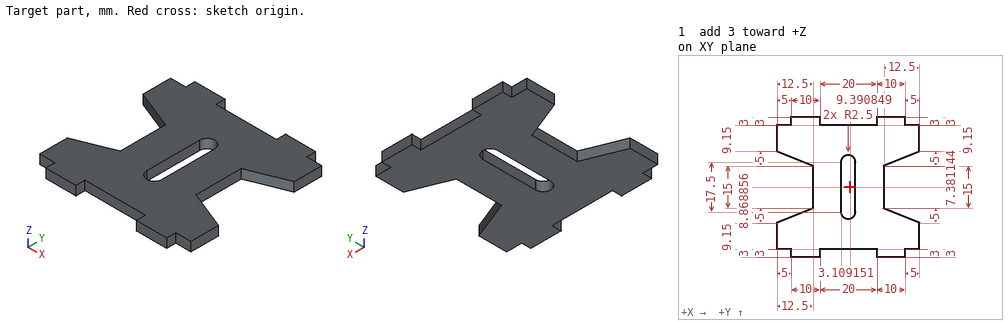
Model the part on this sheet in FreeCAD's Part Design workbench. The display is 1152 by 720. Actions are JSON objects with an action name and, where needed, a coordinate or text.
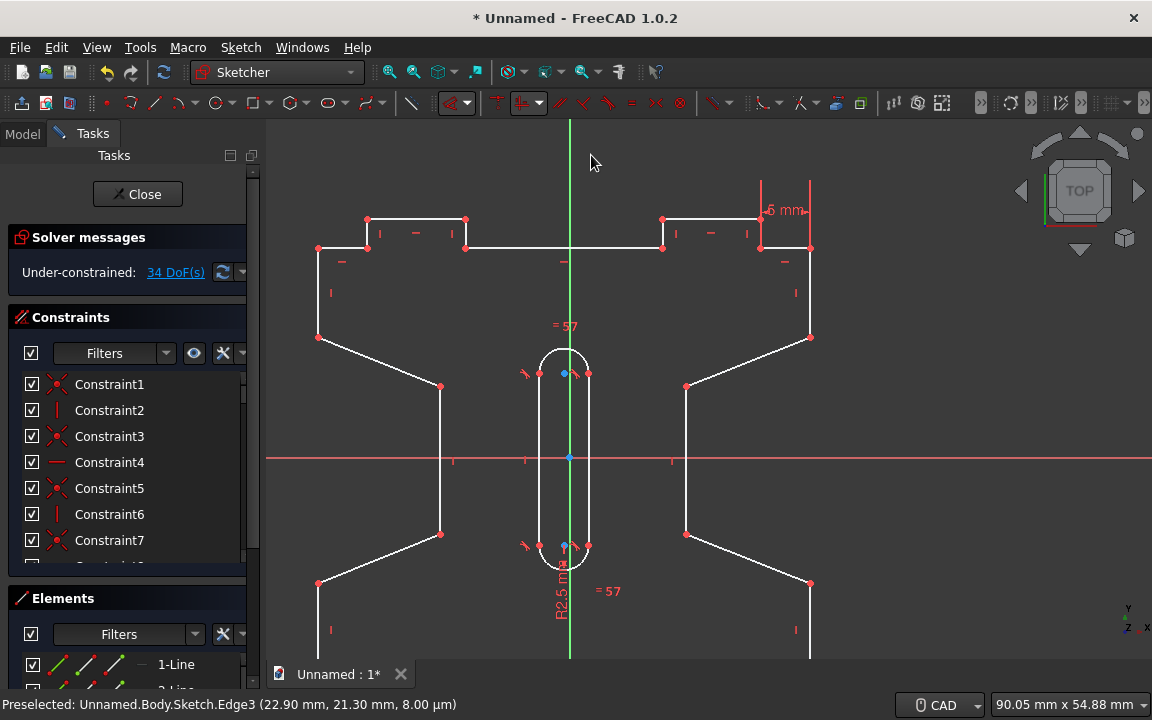
{"action": "scroll", "coordinate": [761, 237], "scroll_direction": "up", "scroll_amount": 2}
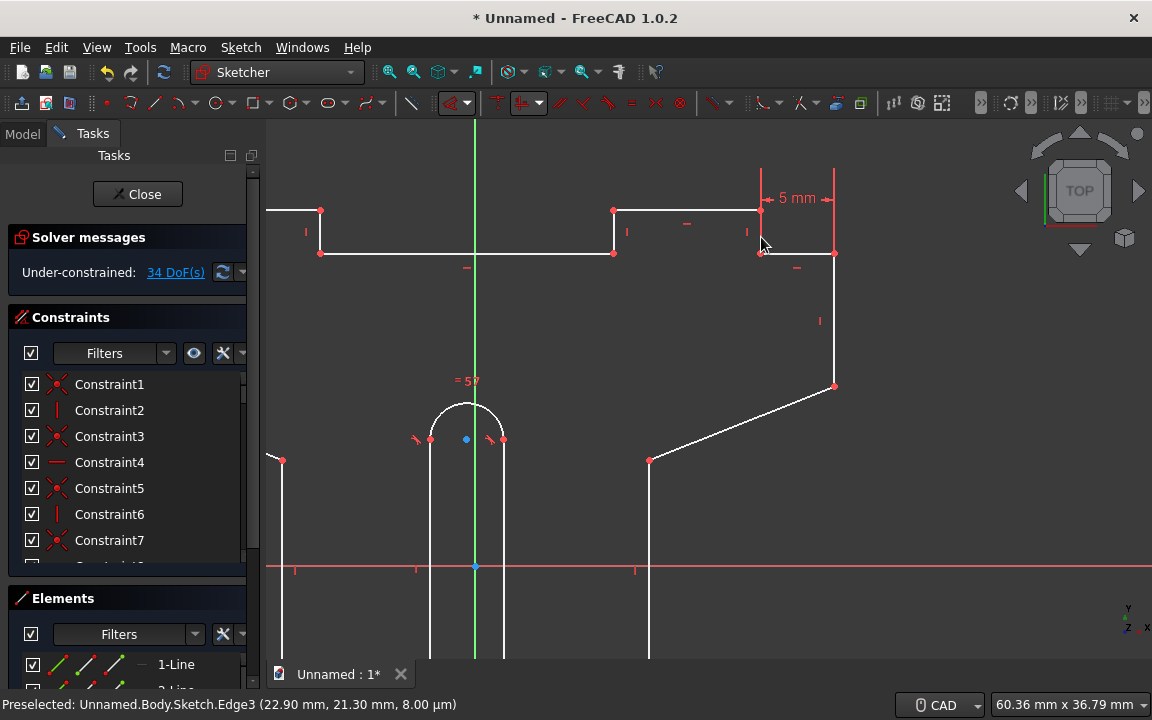
{"action": "left_click", "coordinate": [761, 236]}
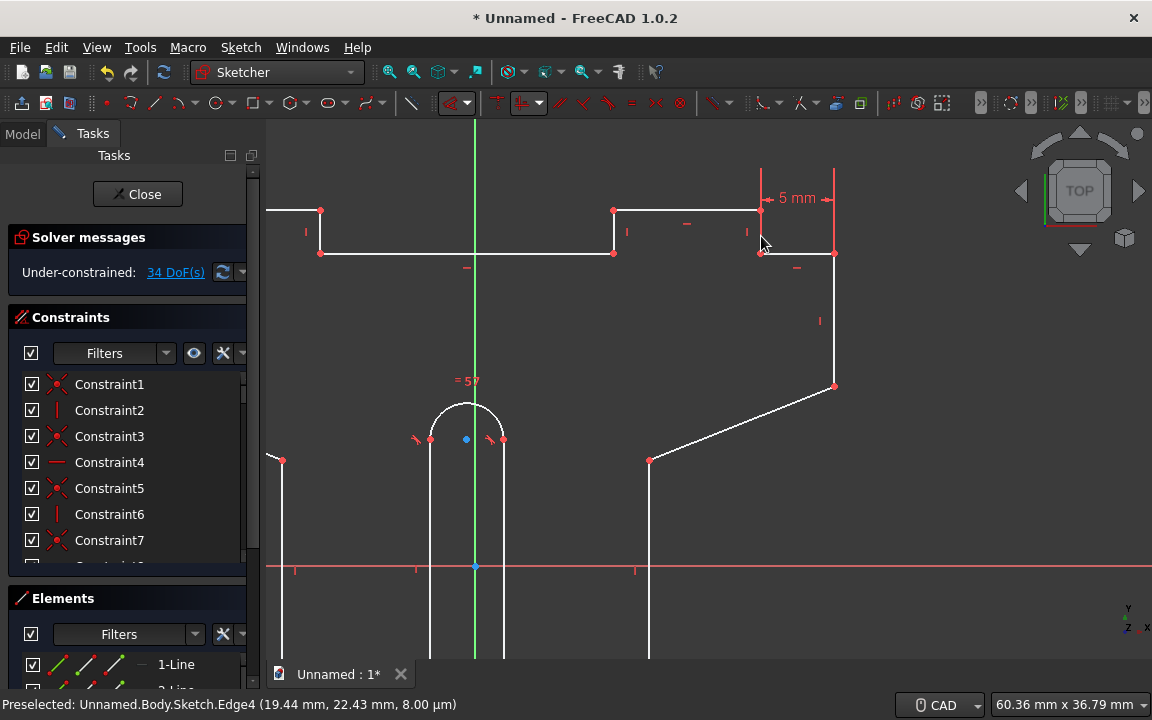
{"action": "left_click", "coordinate": [470, 104]}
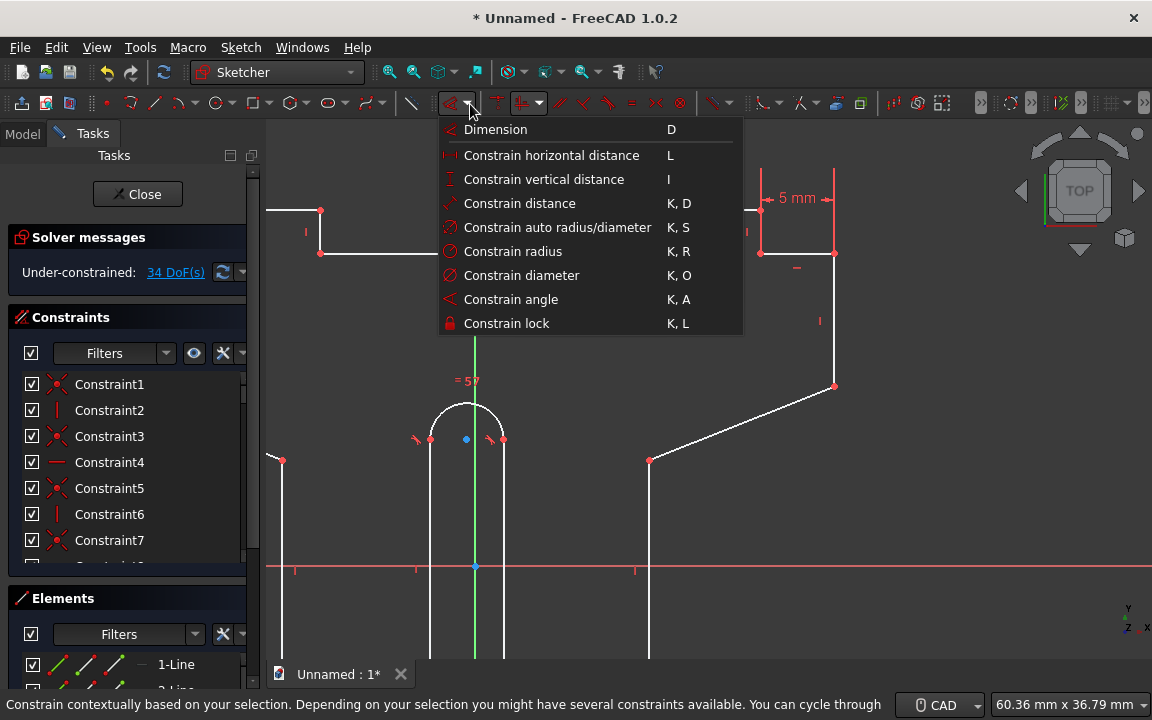
{"action": "left_click", "coordinate": [591, 179]}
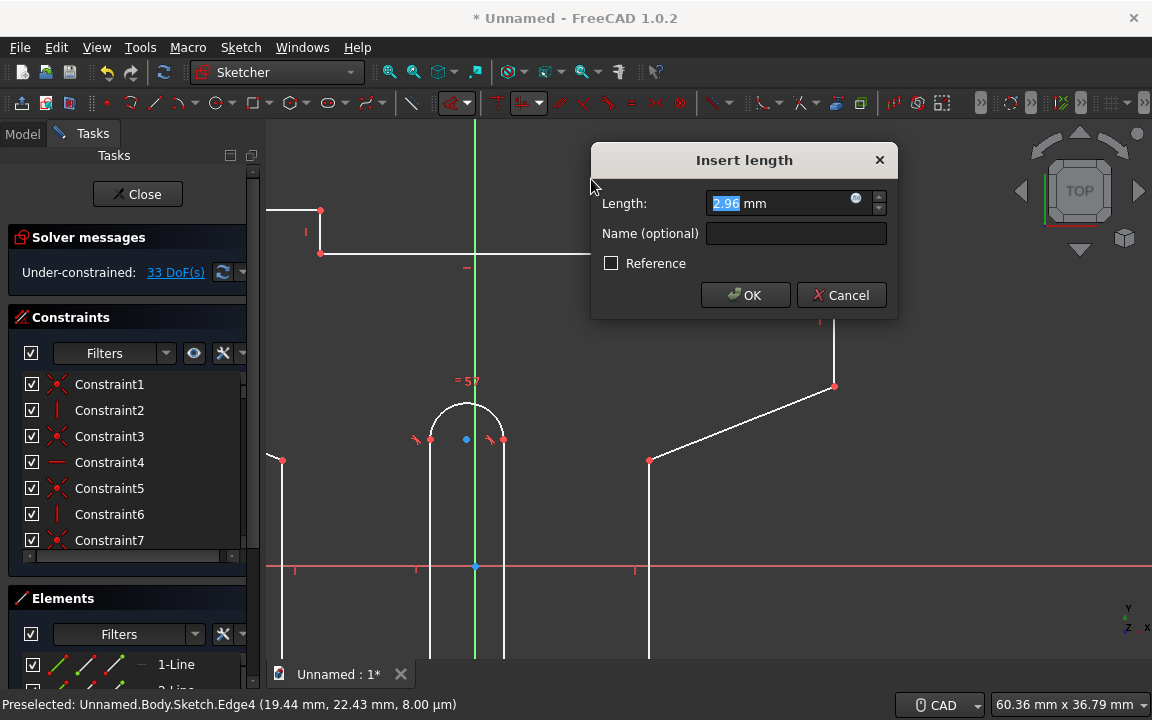
{"action": "type", "text": "3"}
{"action": "key", "text": "Return"}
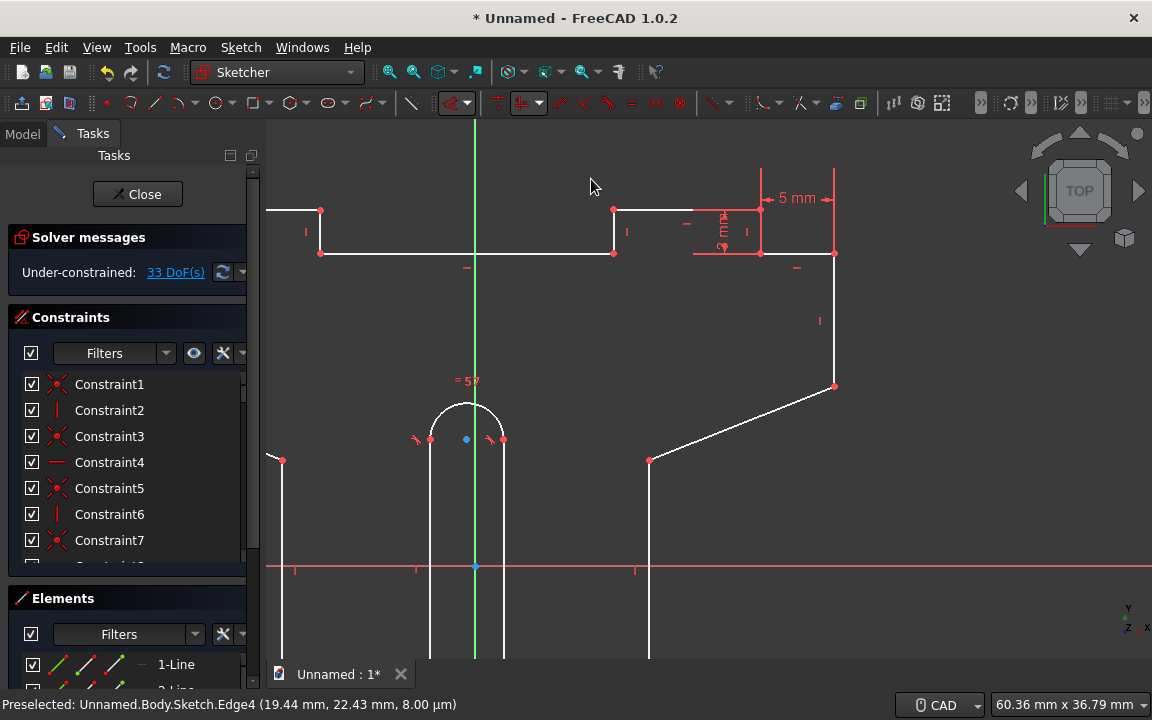
{"action": "left_click", "coordinate": [614, 223]}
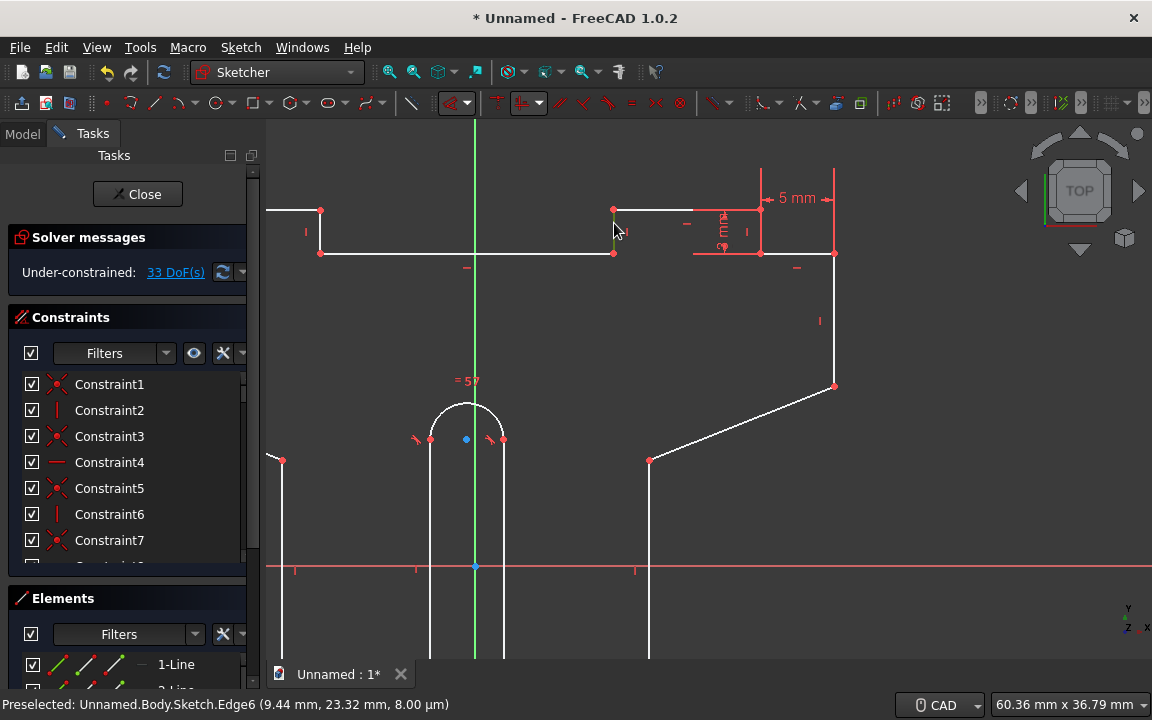
{"action": "key", "text": "i"}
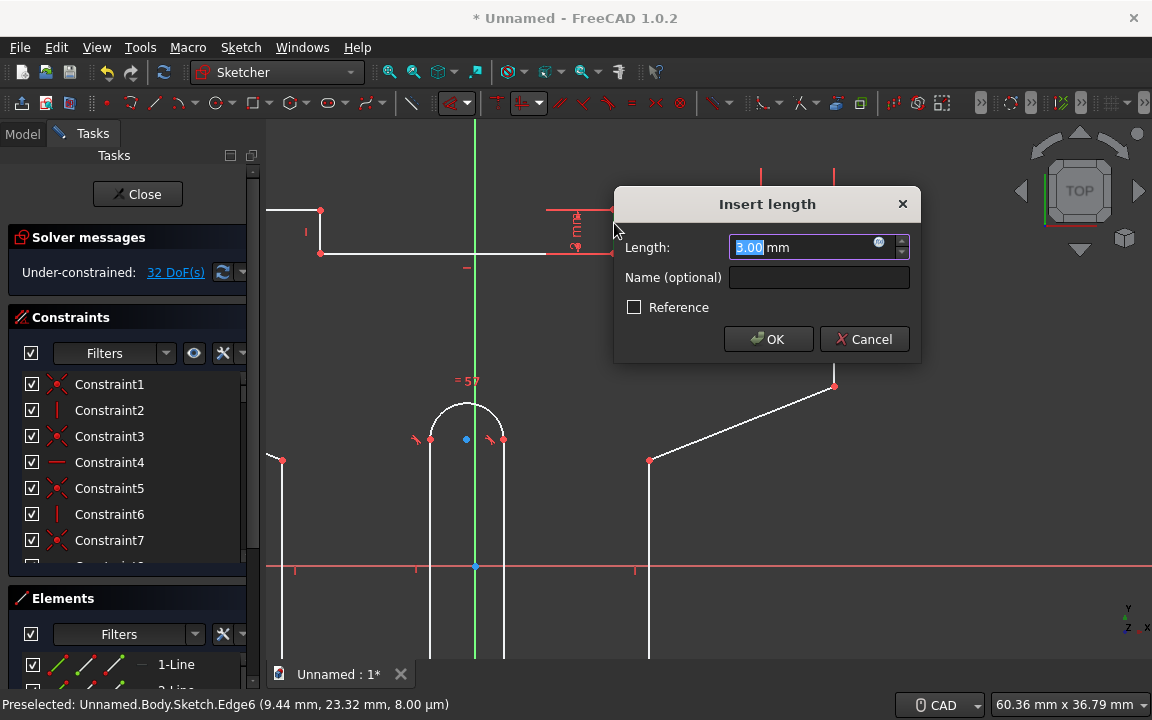
{"action": "type", "text": "3"}
{"action": "key", "text": "Return"}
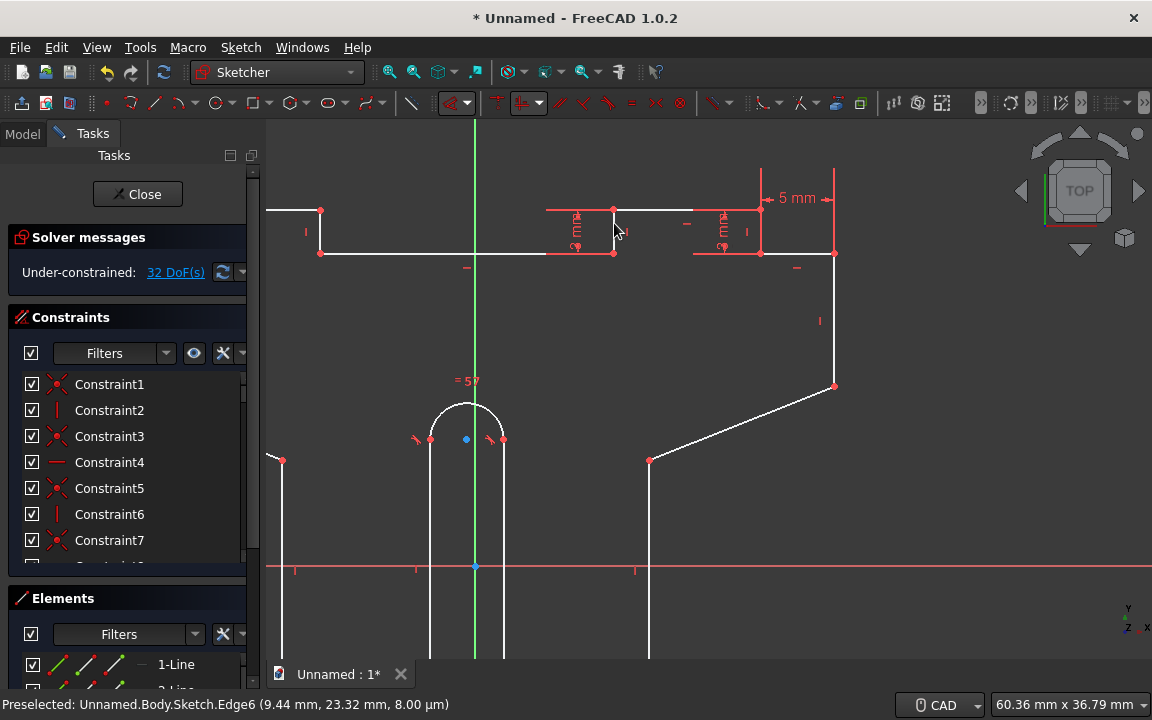
{"action": "left_click", "coordinate": [320, 241]}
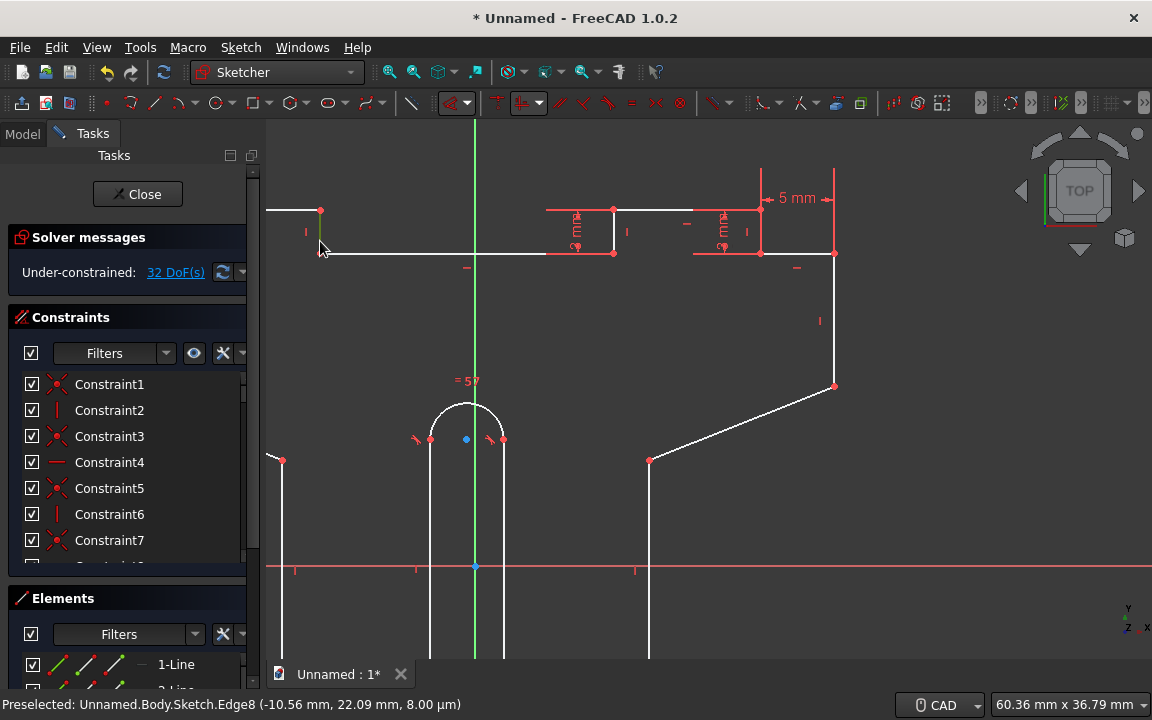
{"action": "key", "text": "i"}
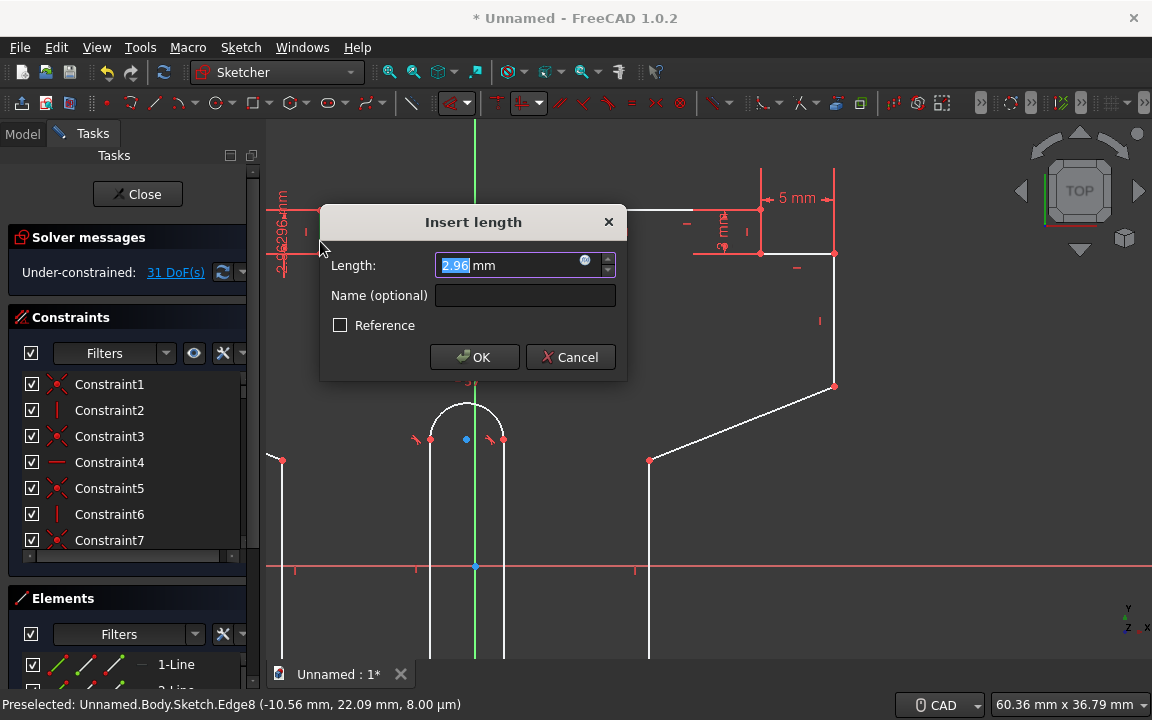
{"action": "type", "text": "3"}
{"action": "key", "text": "Return"}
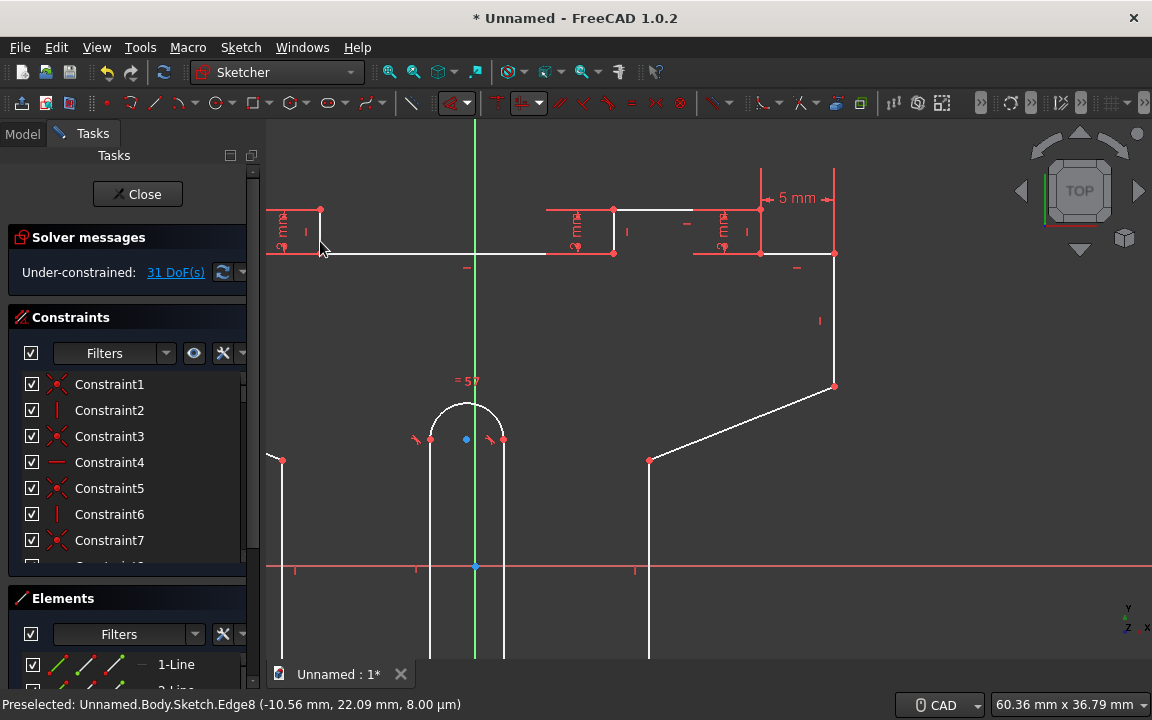
{"action": "scroll", "coordinate": [783, 243], "scroll_direction": "down", "scroll_amount": 4}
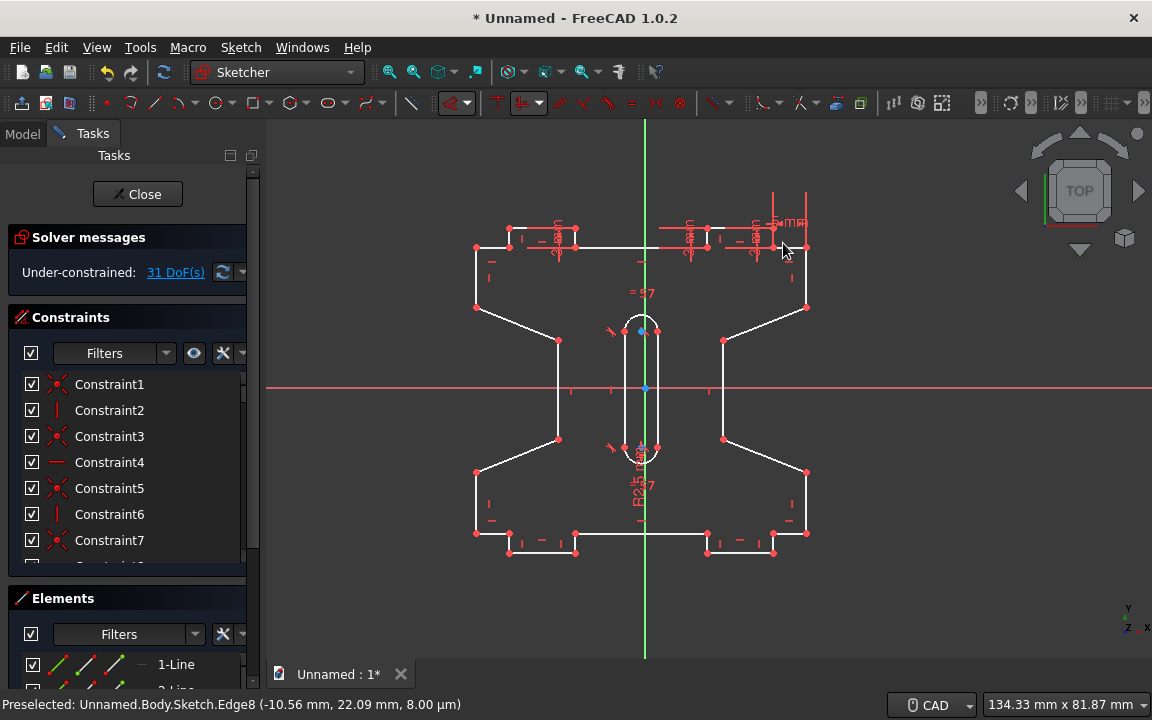
{"action": "scroll", "coordinate": [509, 234], "scroll_direction": "up", "scroll_amount": 5}